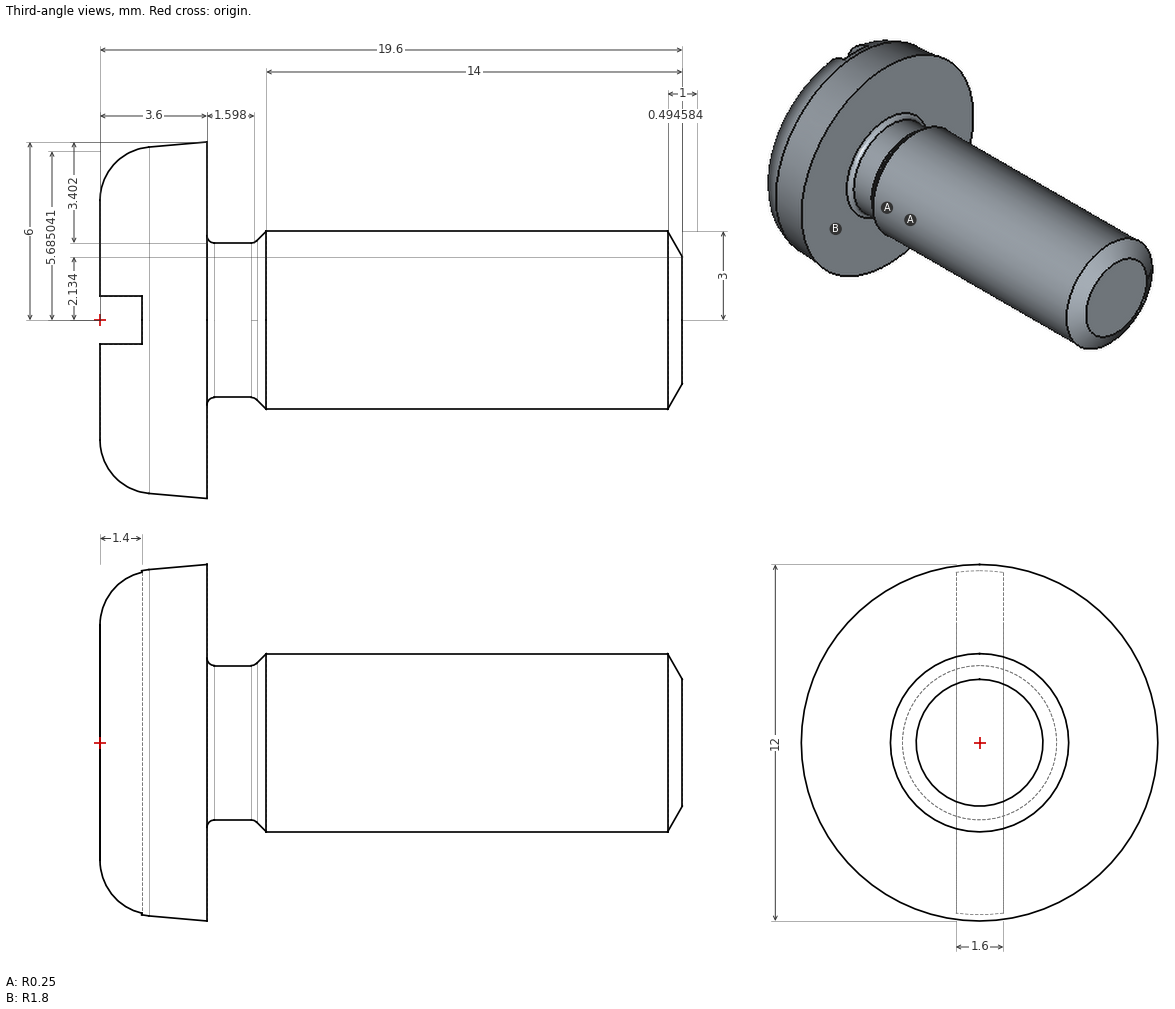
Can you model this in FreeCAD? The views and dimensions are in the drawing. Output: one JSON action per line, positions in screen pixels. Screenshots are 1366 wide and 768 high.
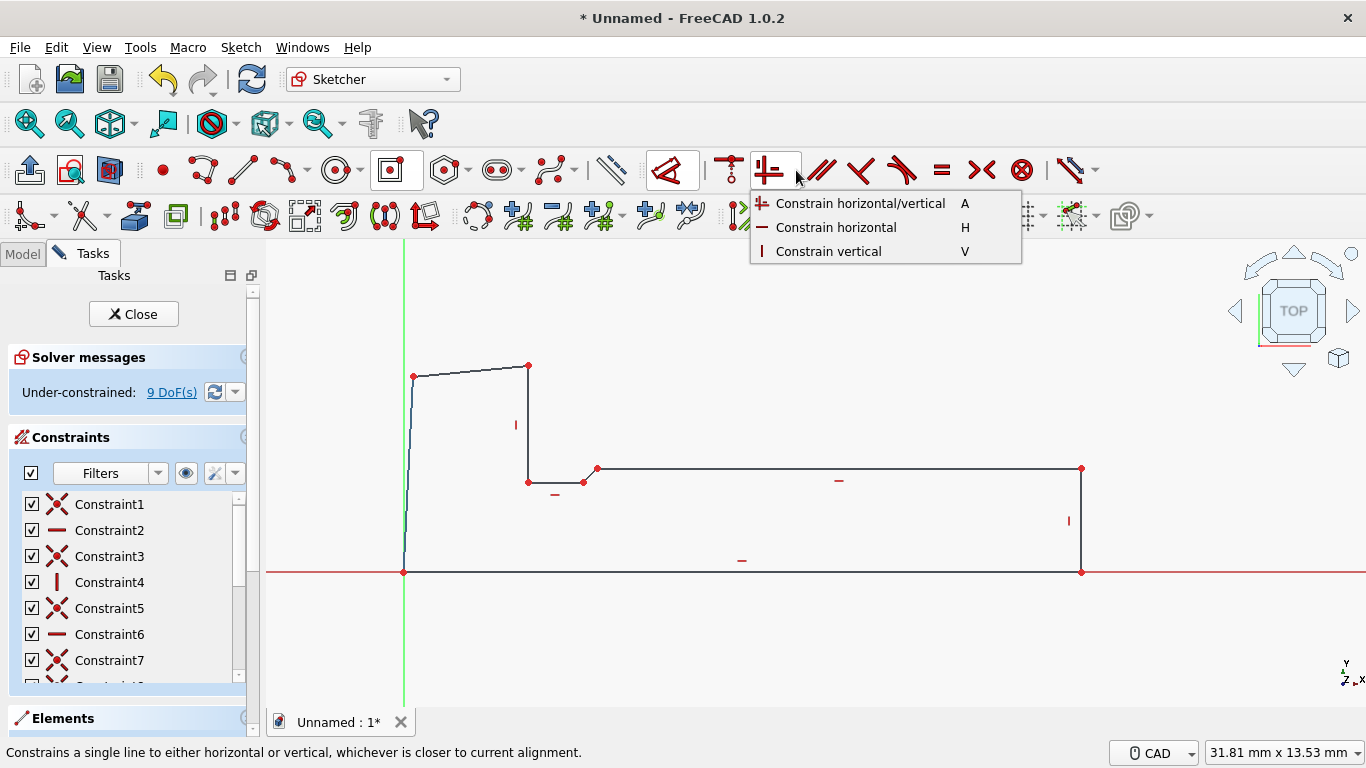
{"action": "left_click", "coordinate": [886, 251]}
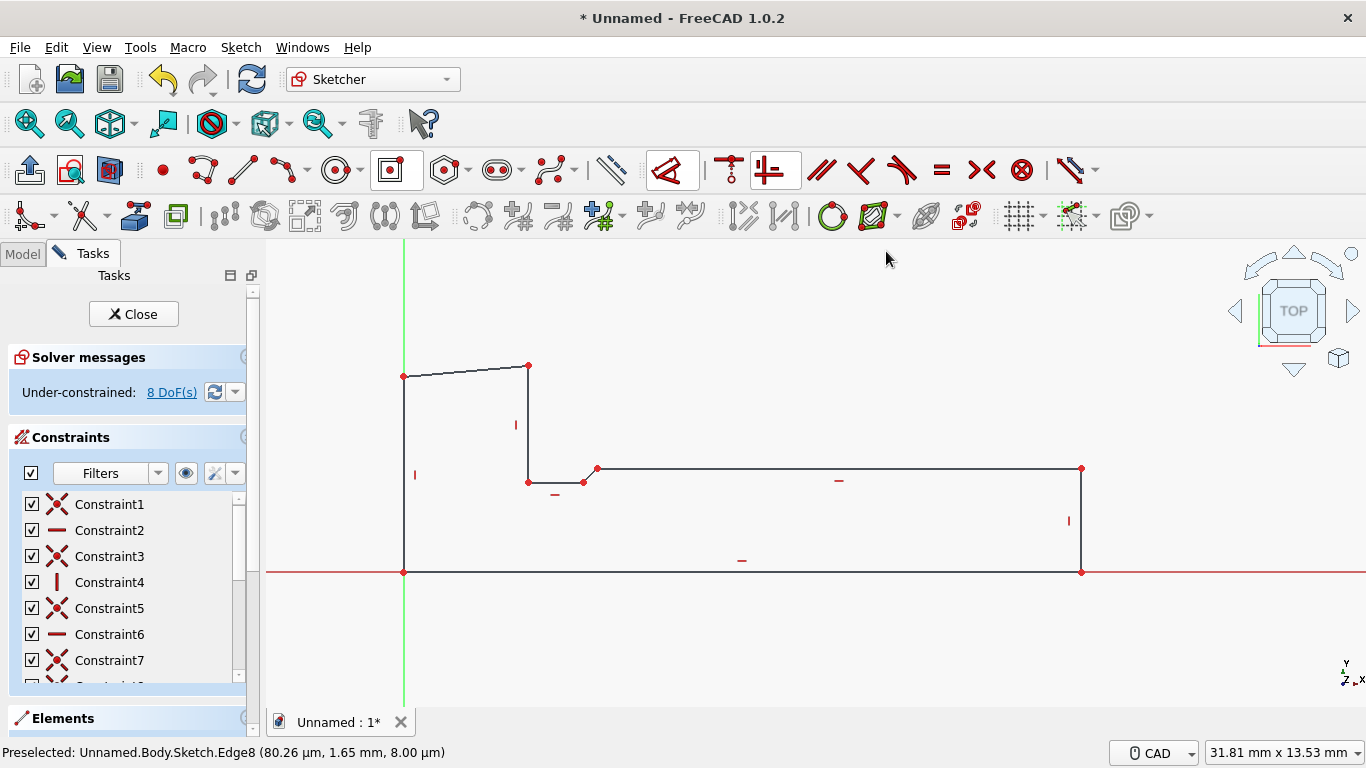
{"action": "left_click", "coordinate": [666, 170]}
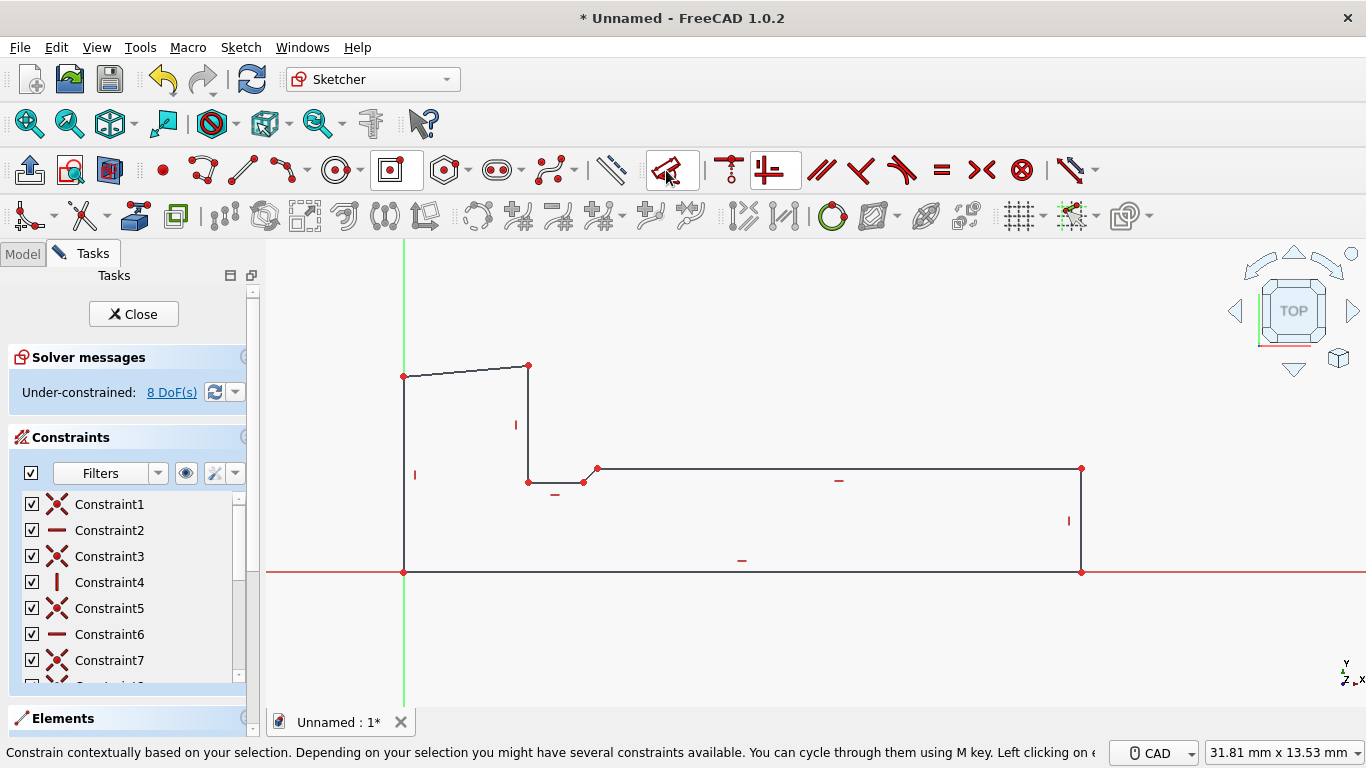
{"action": "left_click", "coordinate": [1081, 541]}
{"action": "left_click", "coordinate": [1115, 521]}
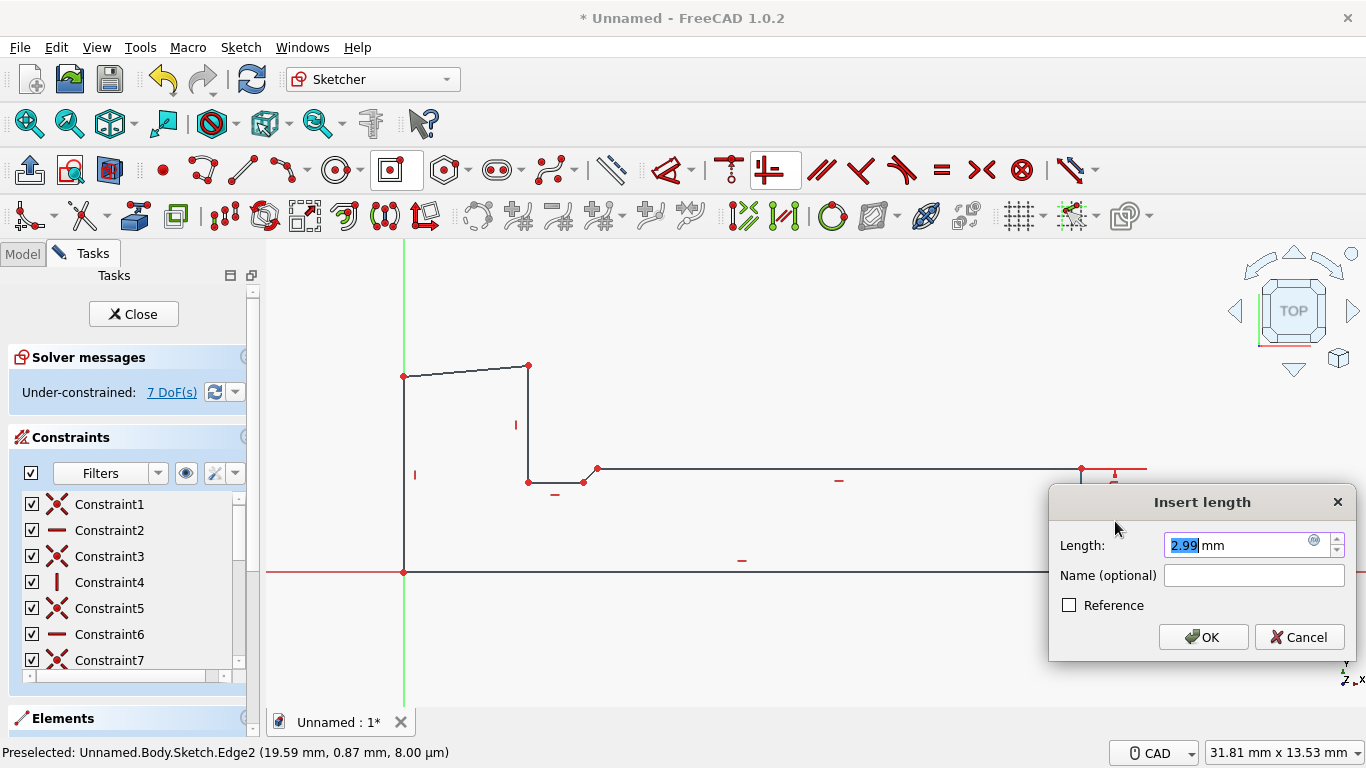
{"action": "type", "text": "3"}
{"action": "key", "text": "Return"}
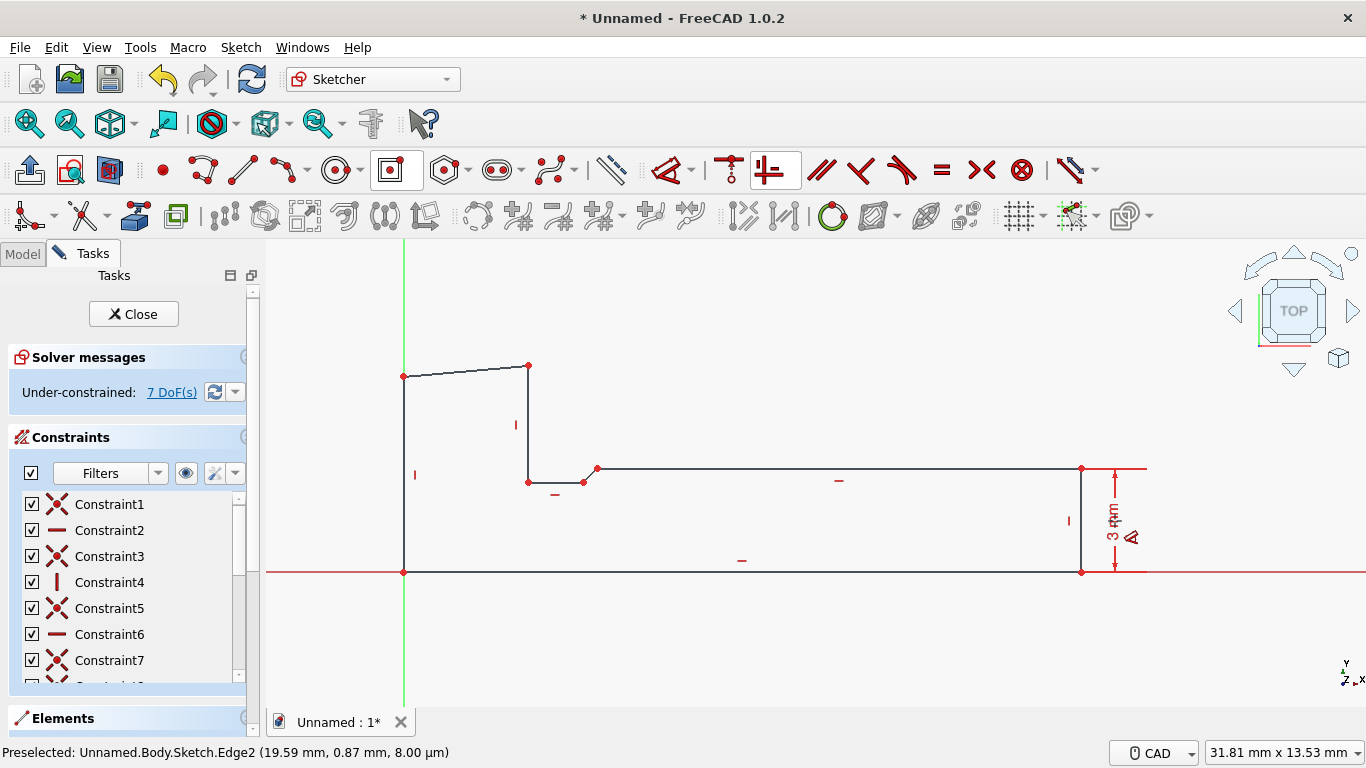
{"action": "left_click", "coordinate": [936, 468]}
{"action": "left_click", "coordinate": [839, 502]}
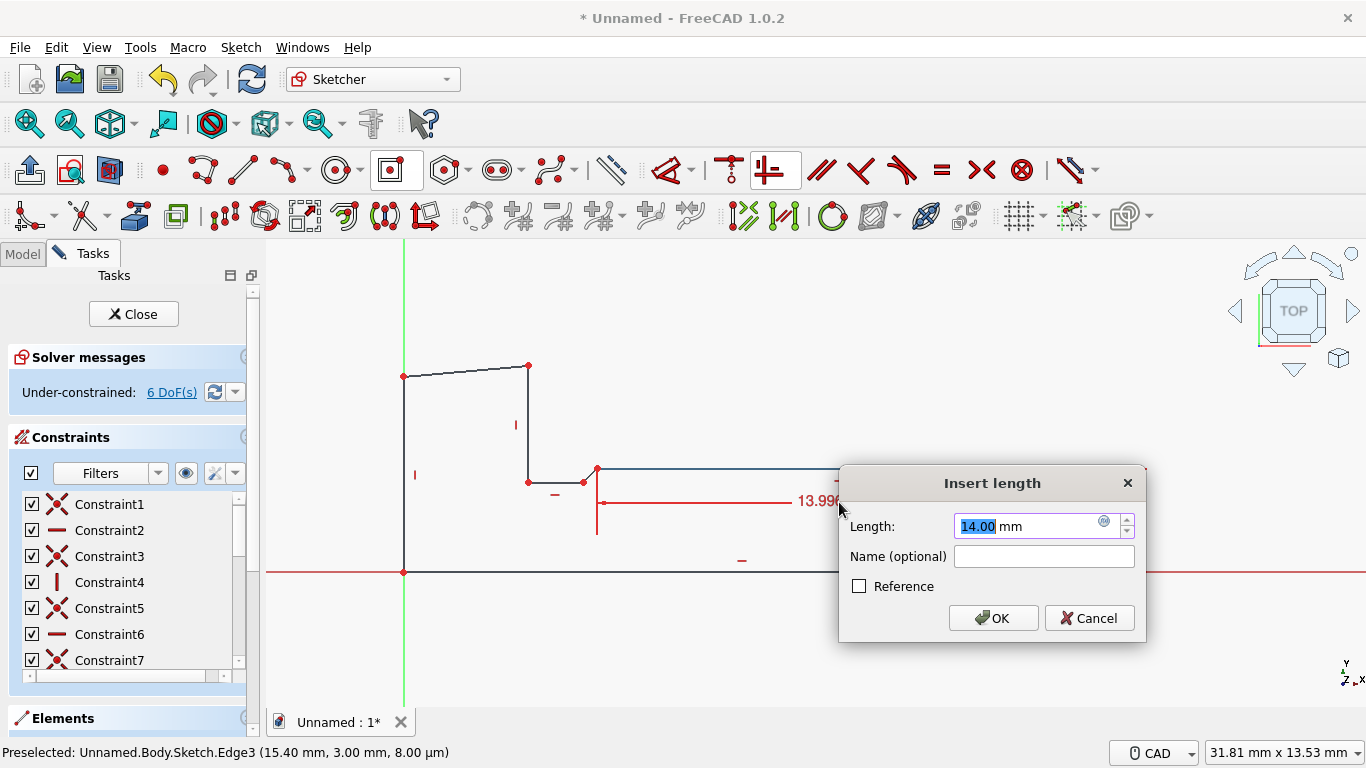
{"action": "type", "text": "14"}
{"action": "key", "text": "Return"}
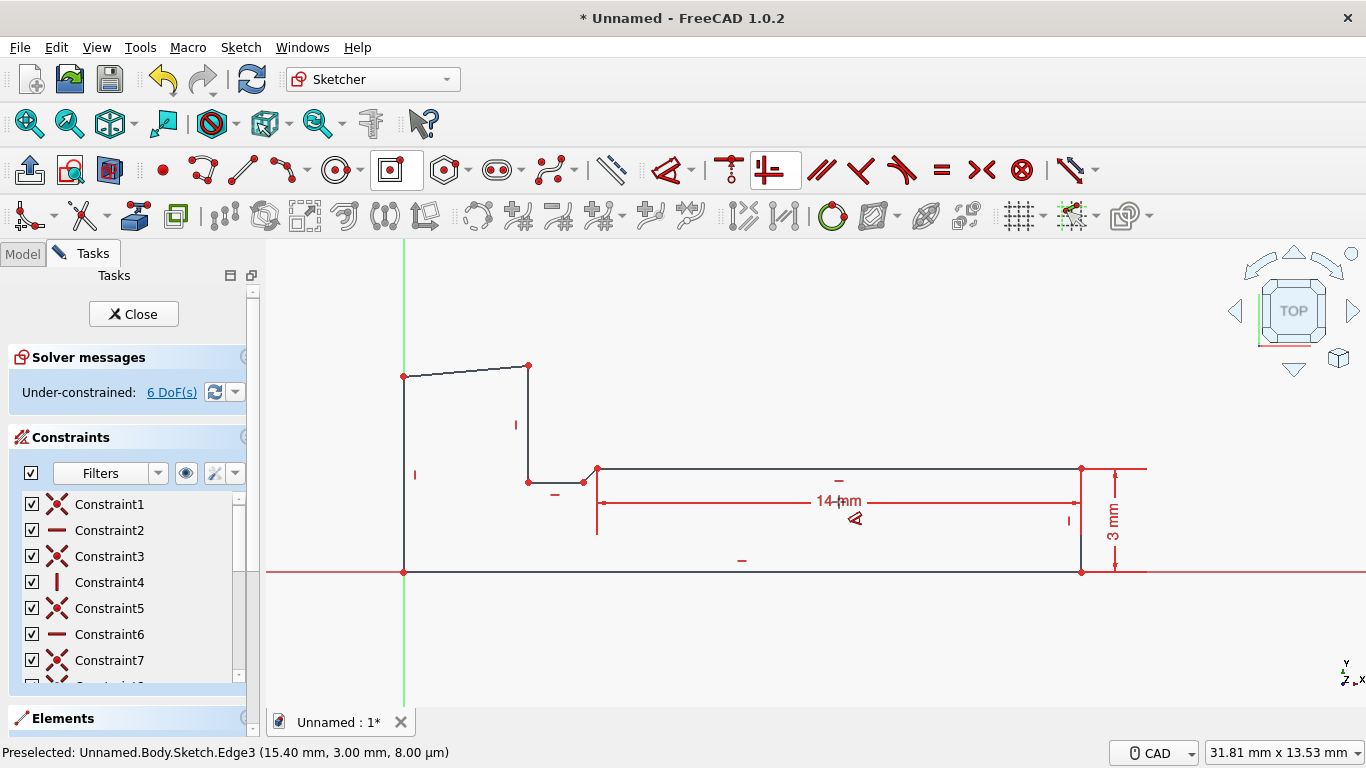
{"action": "left_click", "coordinate": [528, 366]}
{"action": "left_click", "coordinate": [370, 469]}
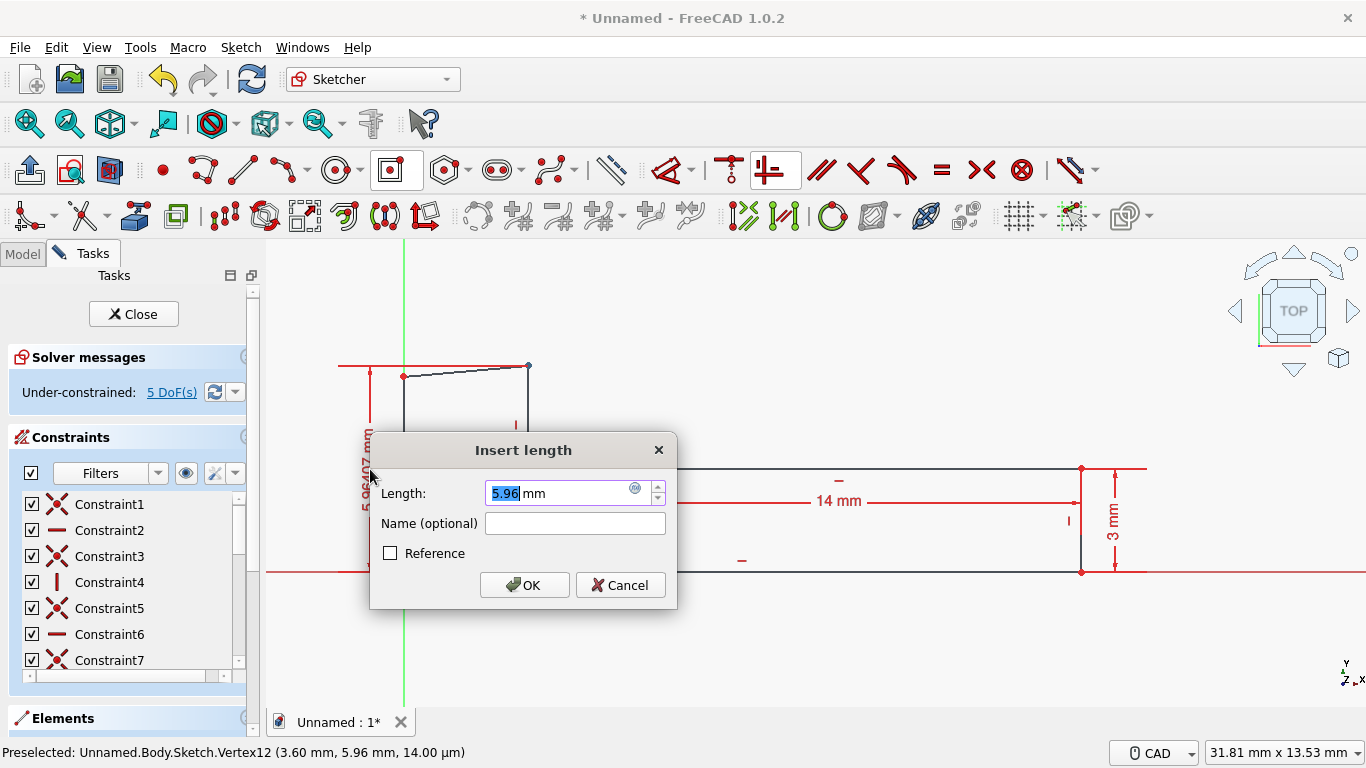
{"action": "type", "text": "6"}
{"action": "key", "text": "Return"}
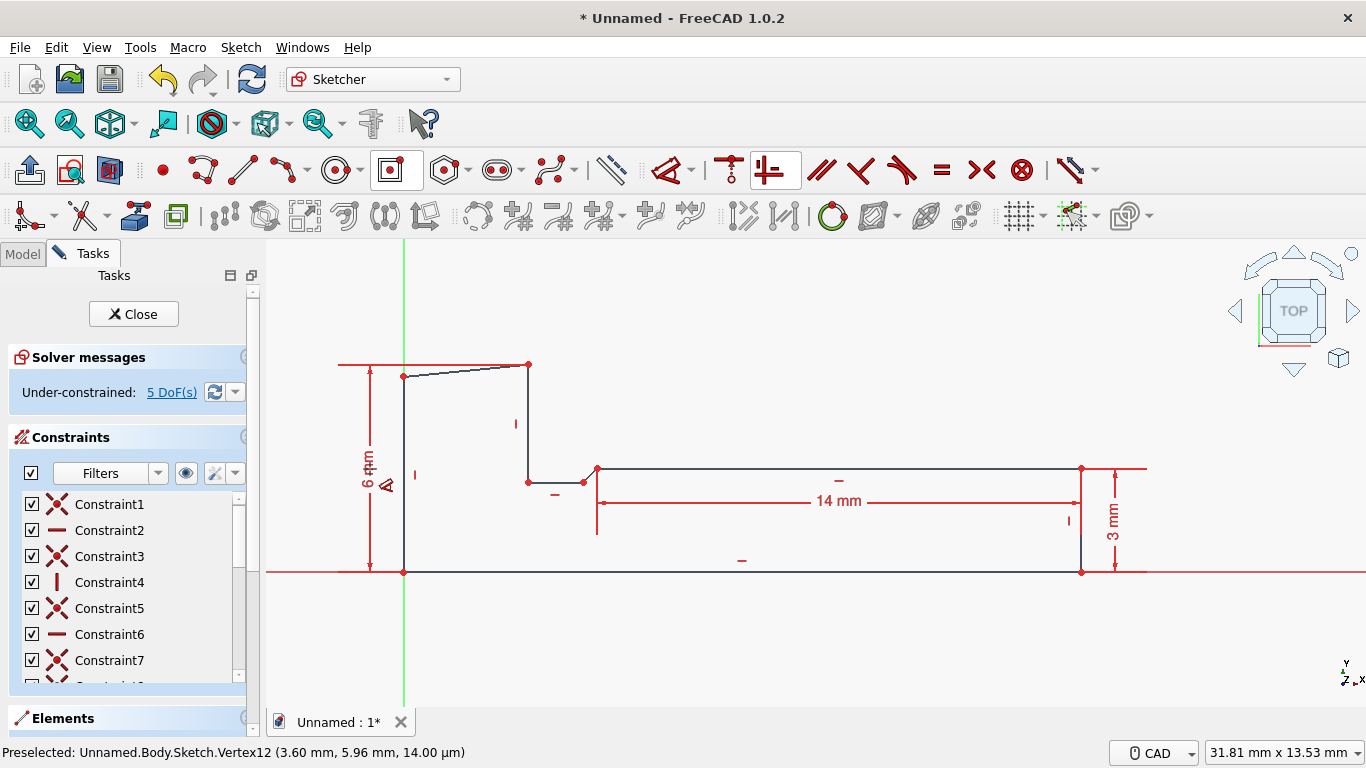
{"action": "left_click", "coordinate": [607, 572]}
{"action": "left_click", "coordinate": [742, 606]}